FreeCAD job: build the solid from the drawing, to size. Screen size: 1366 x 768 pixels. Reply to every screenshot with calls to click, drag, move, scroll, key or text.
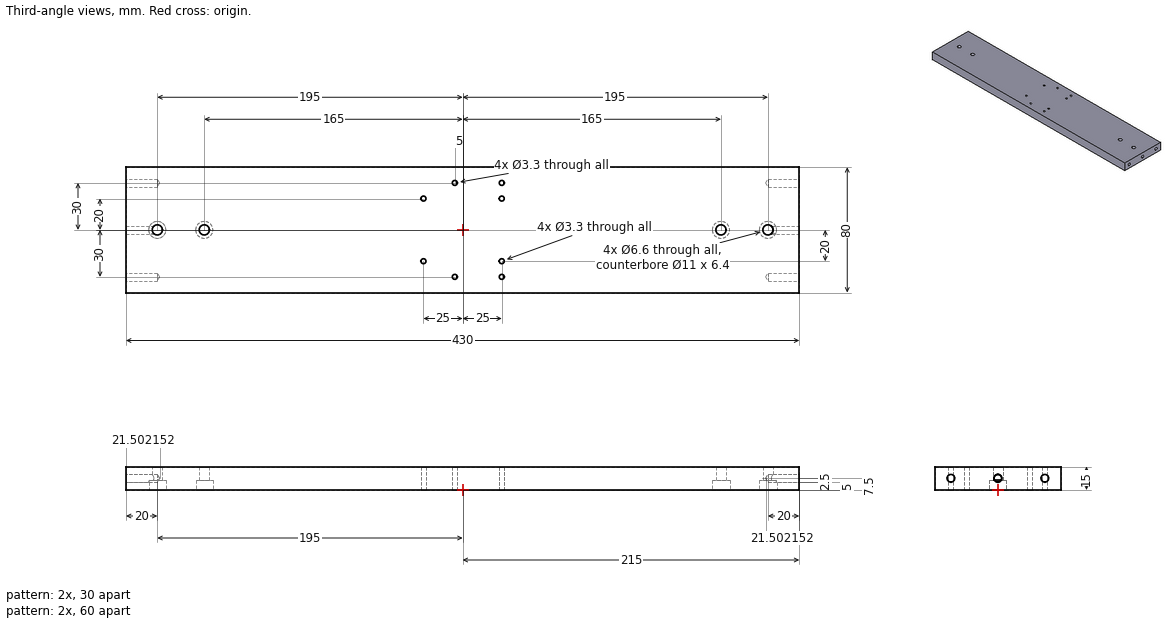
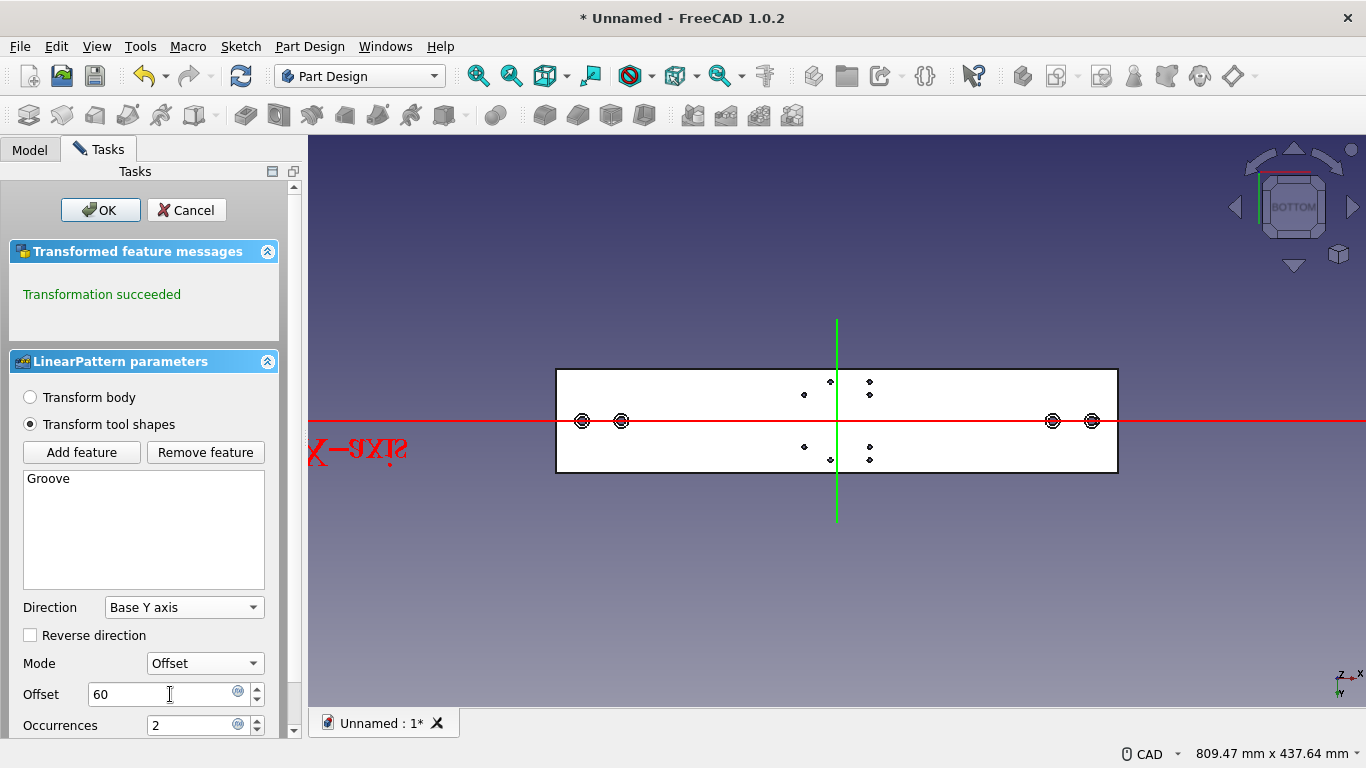
triple_click(199, 726)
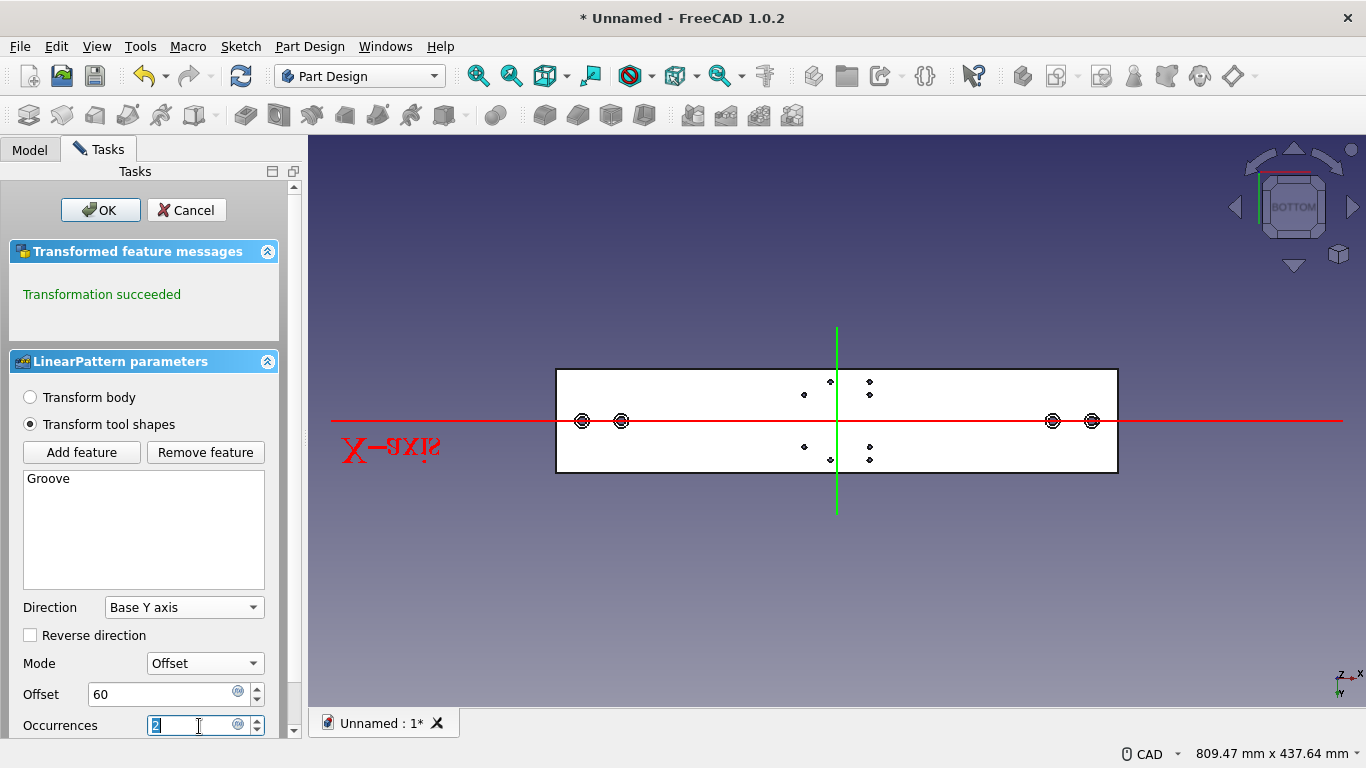
text(2)
key(Tab)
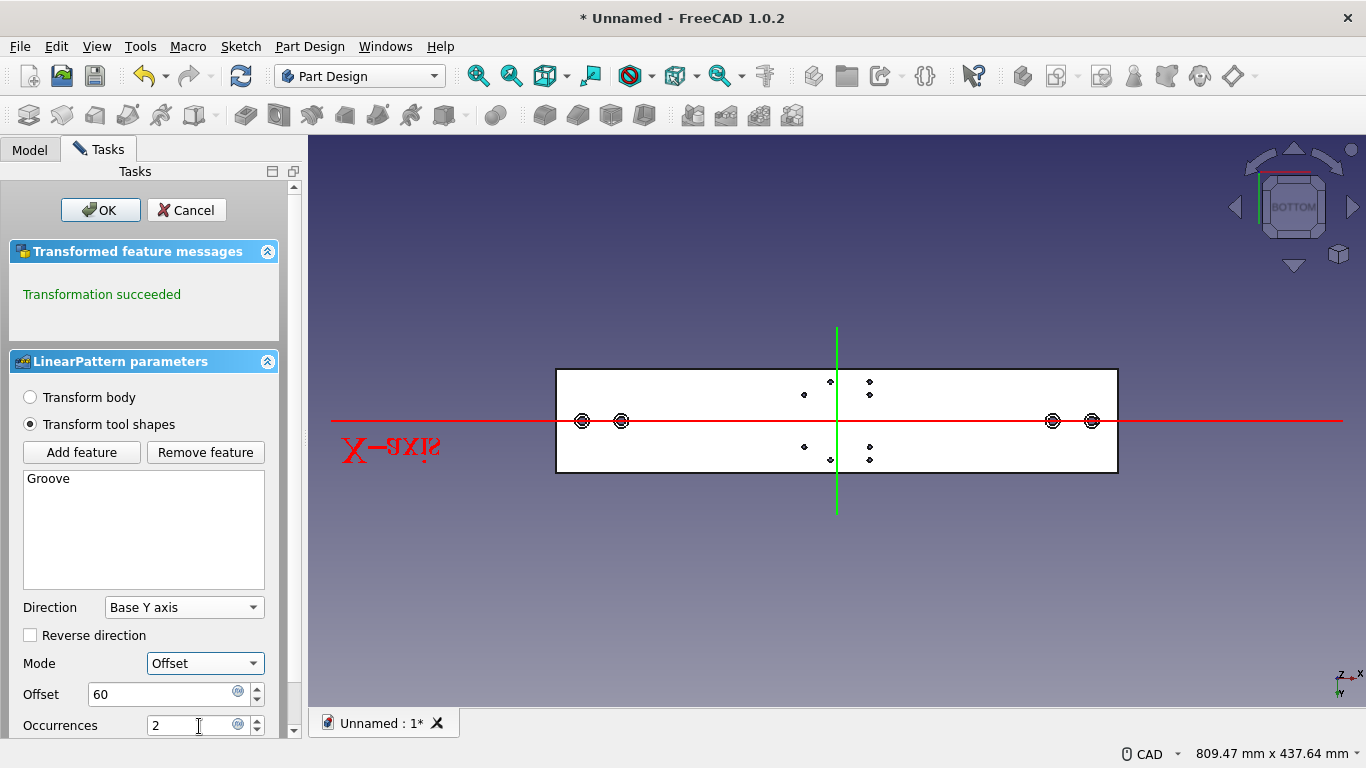
click(31, 635)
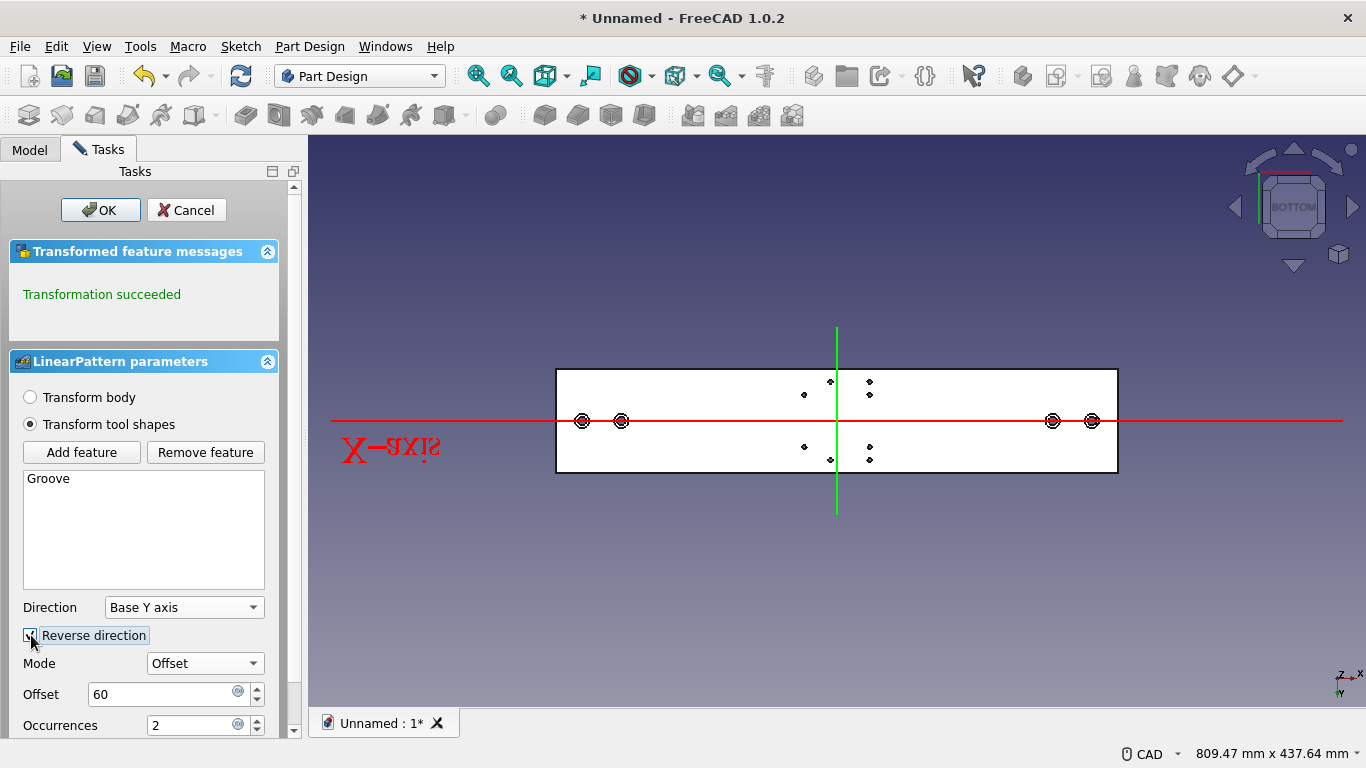
click(101, 210)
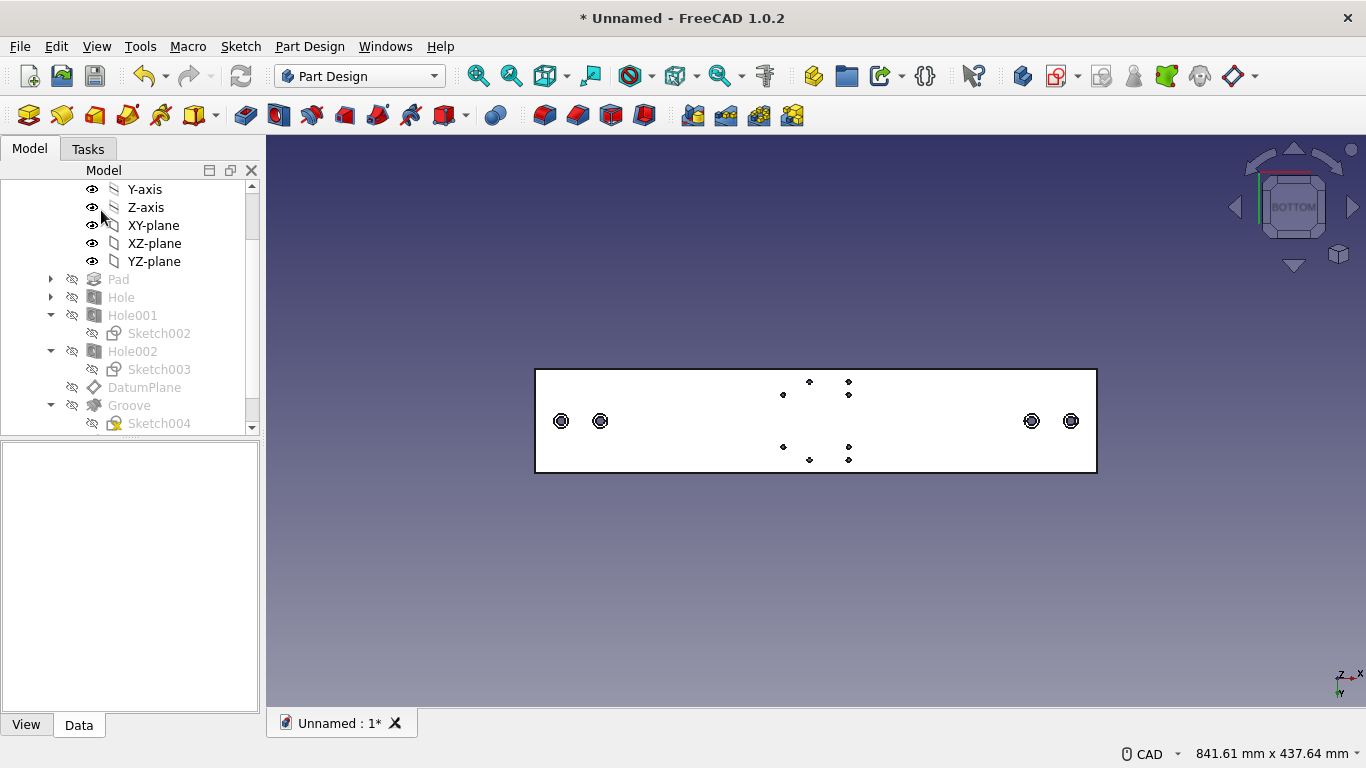
click(117, 405)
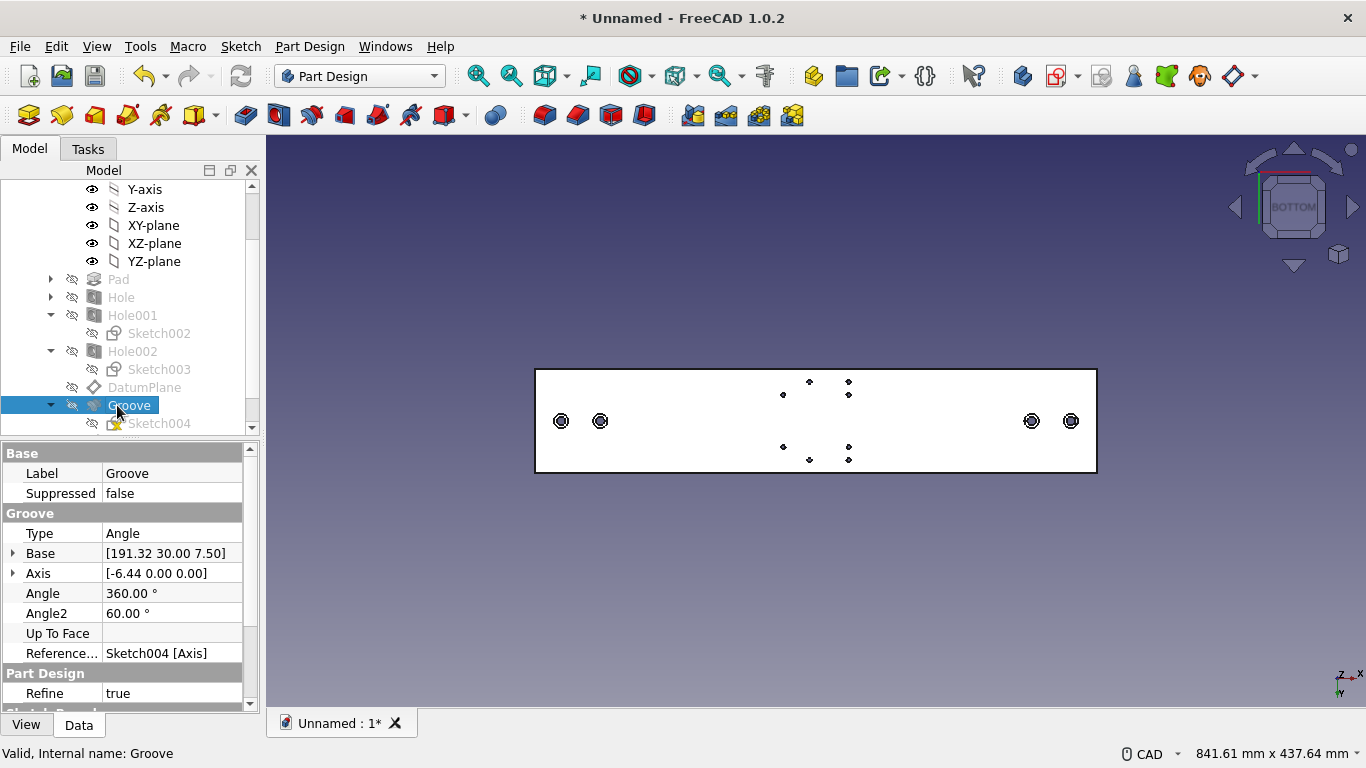
click(693, 116)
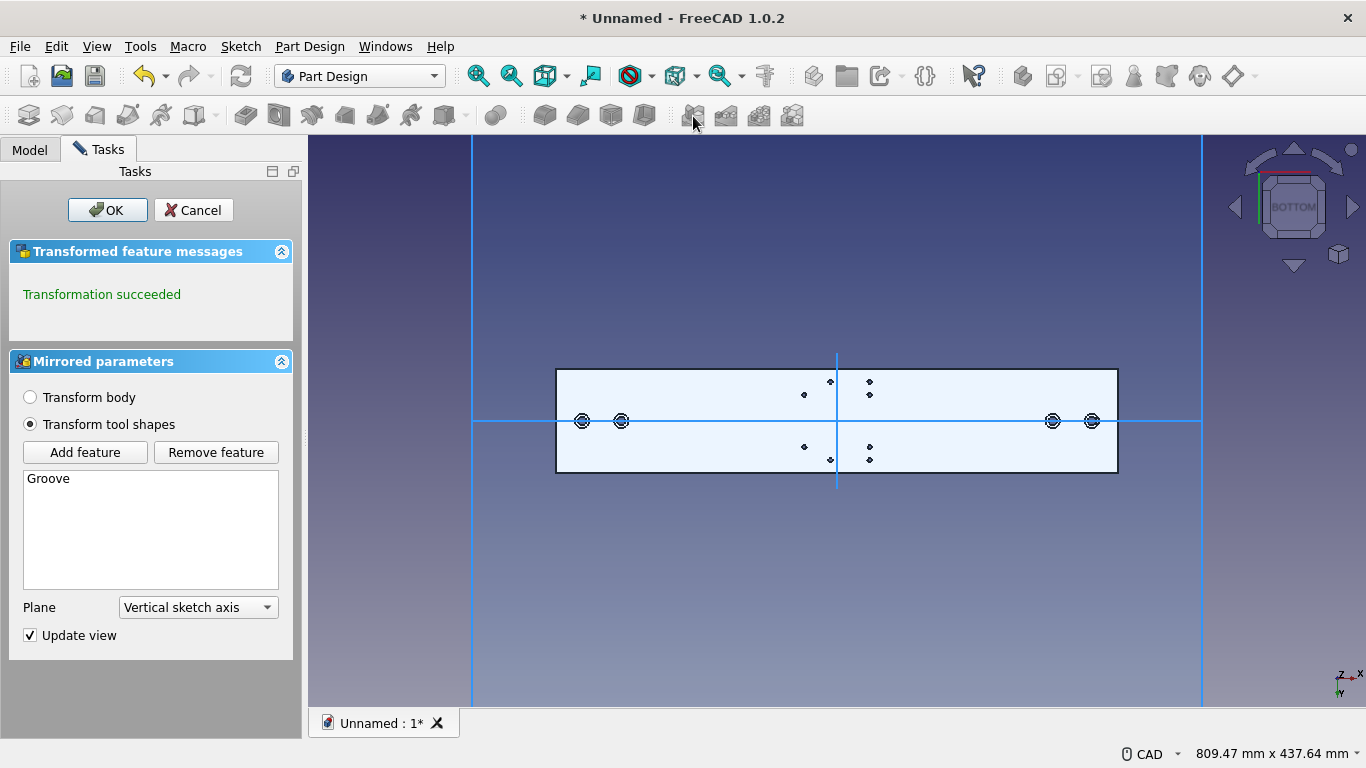
click(199, 608)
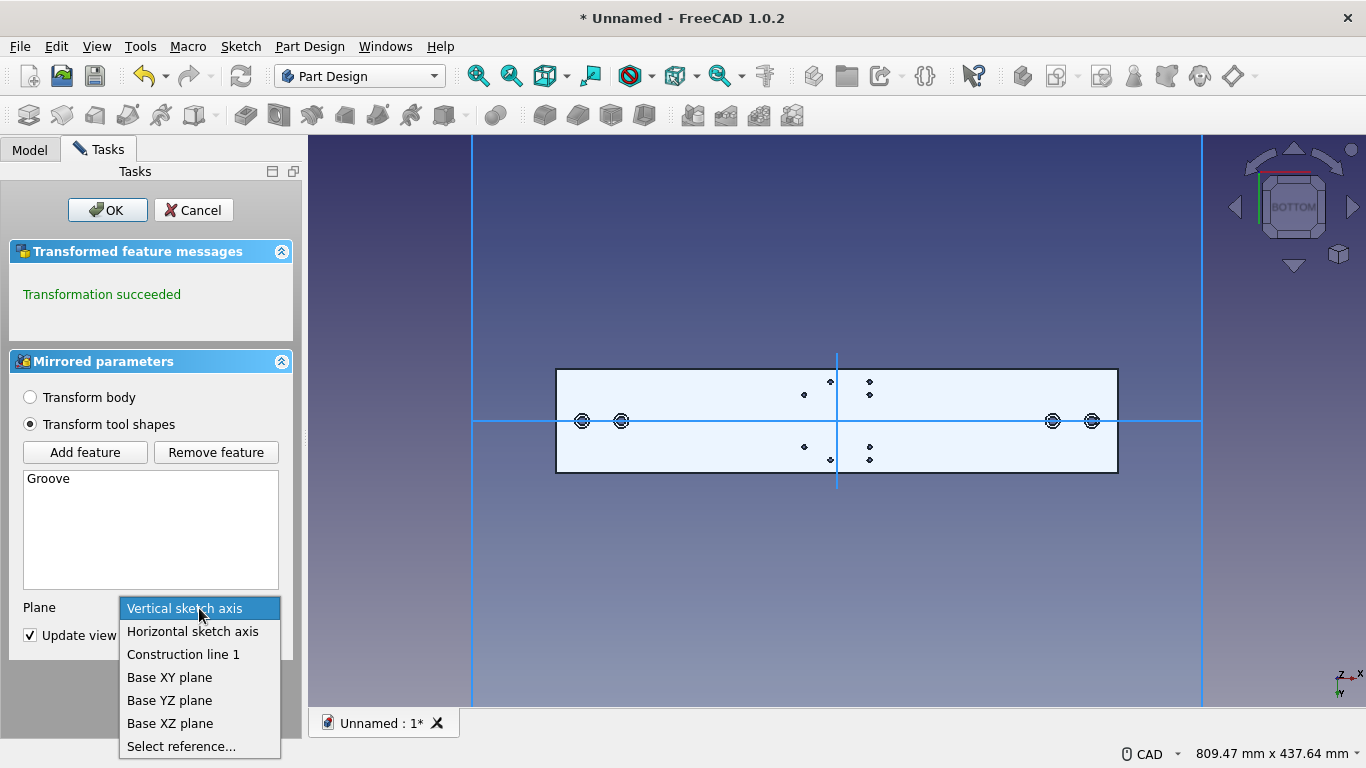
click(198, 700)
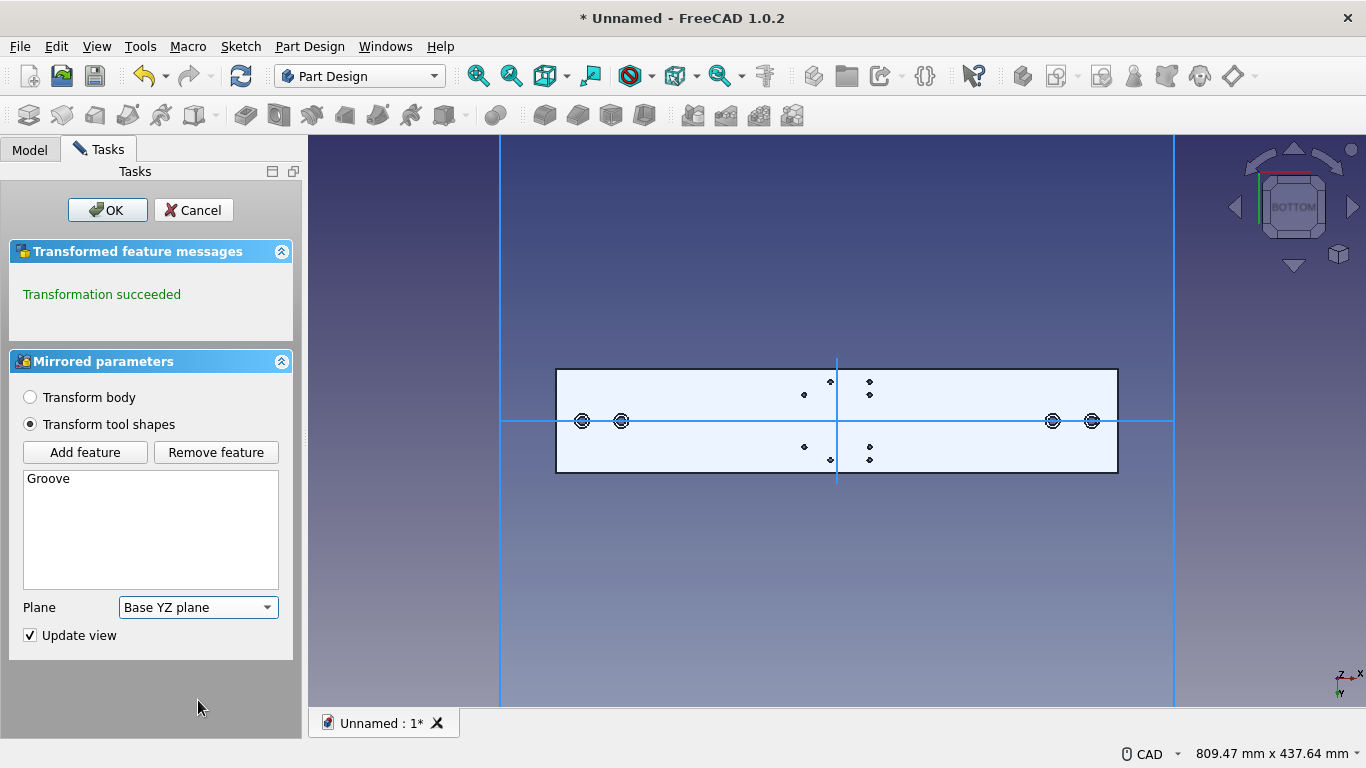
click(108, 210)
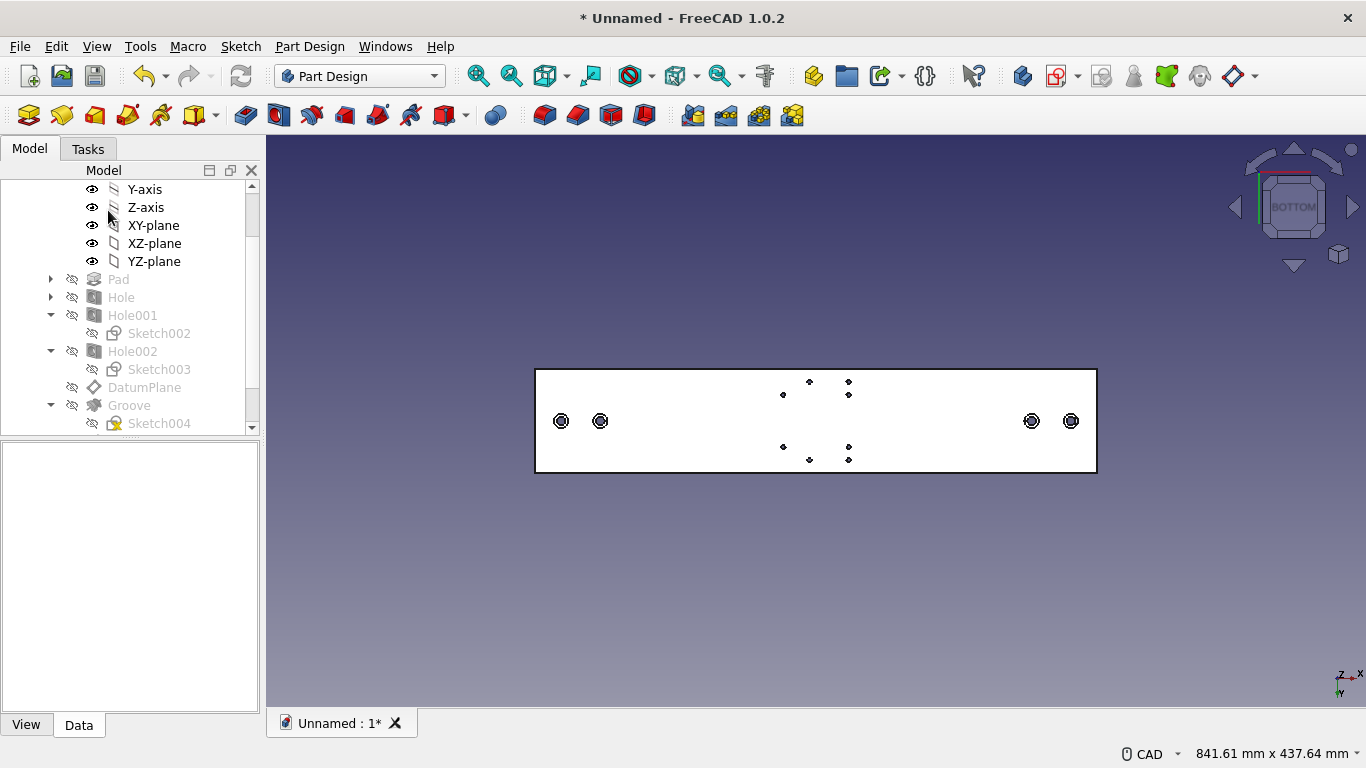
click(1056, 76)